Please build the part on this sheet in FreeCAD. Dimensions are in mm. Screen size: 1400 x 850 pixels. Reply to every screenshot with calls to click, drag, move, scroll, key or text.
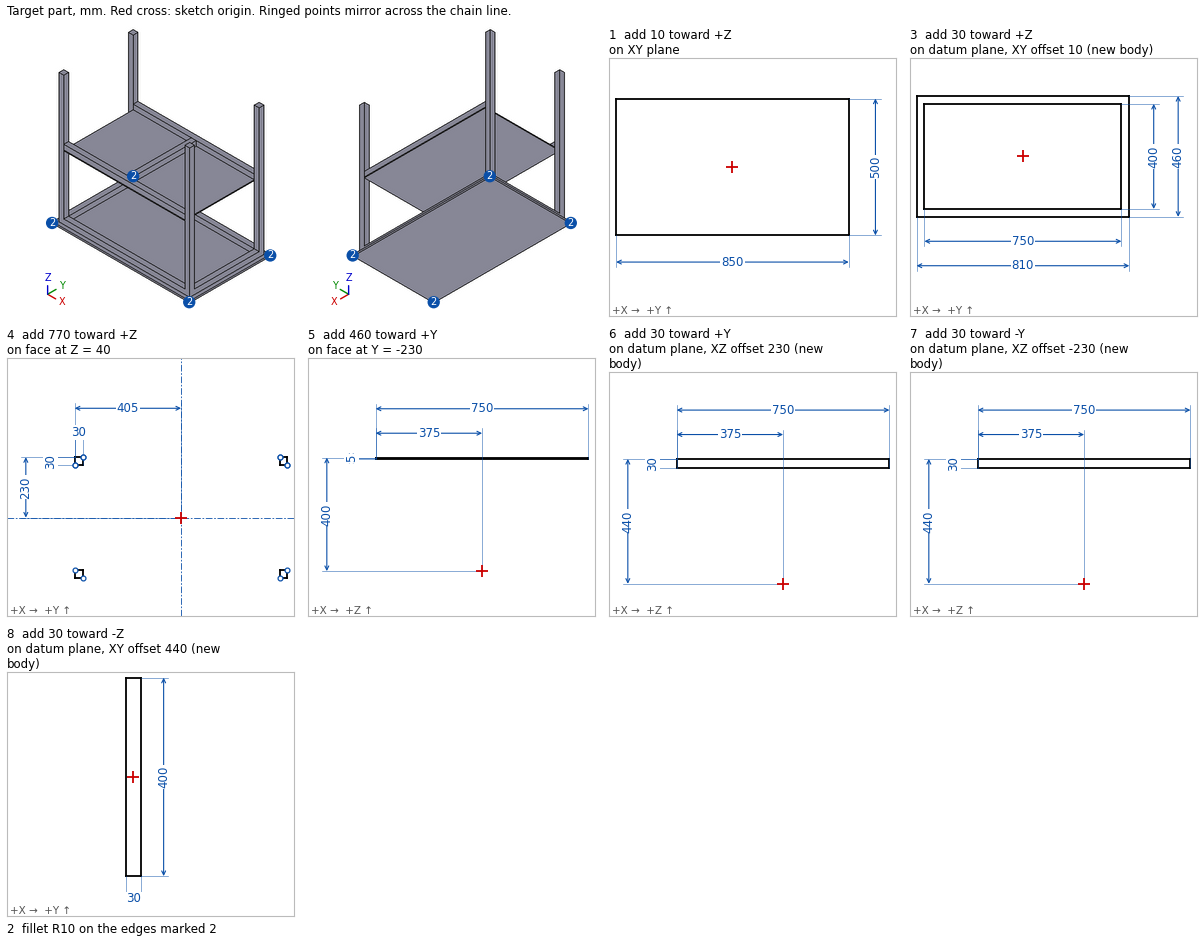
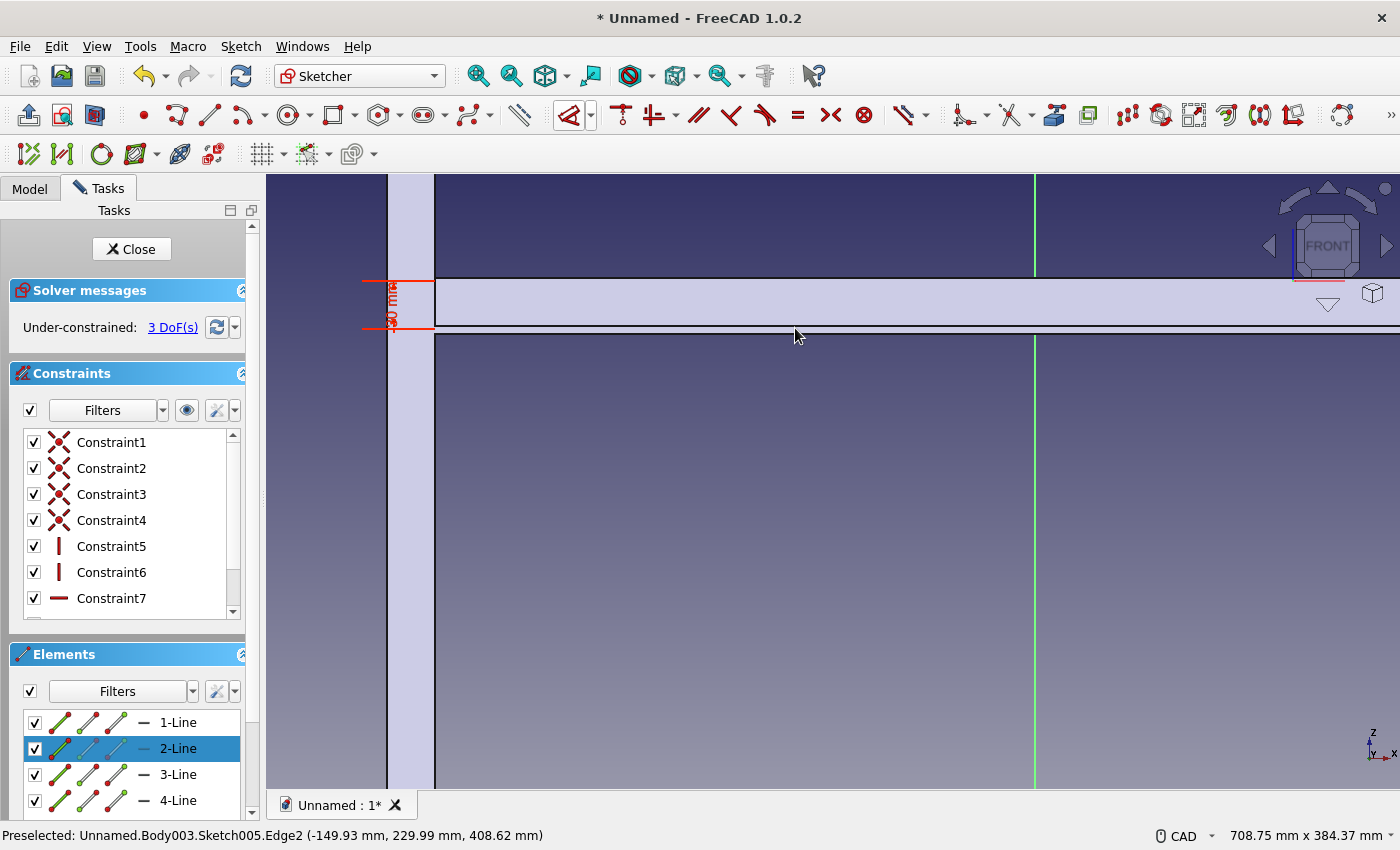
click(590, 116)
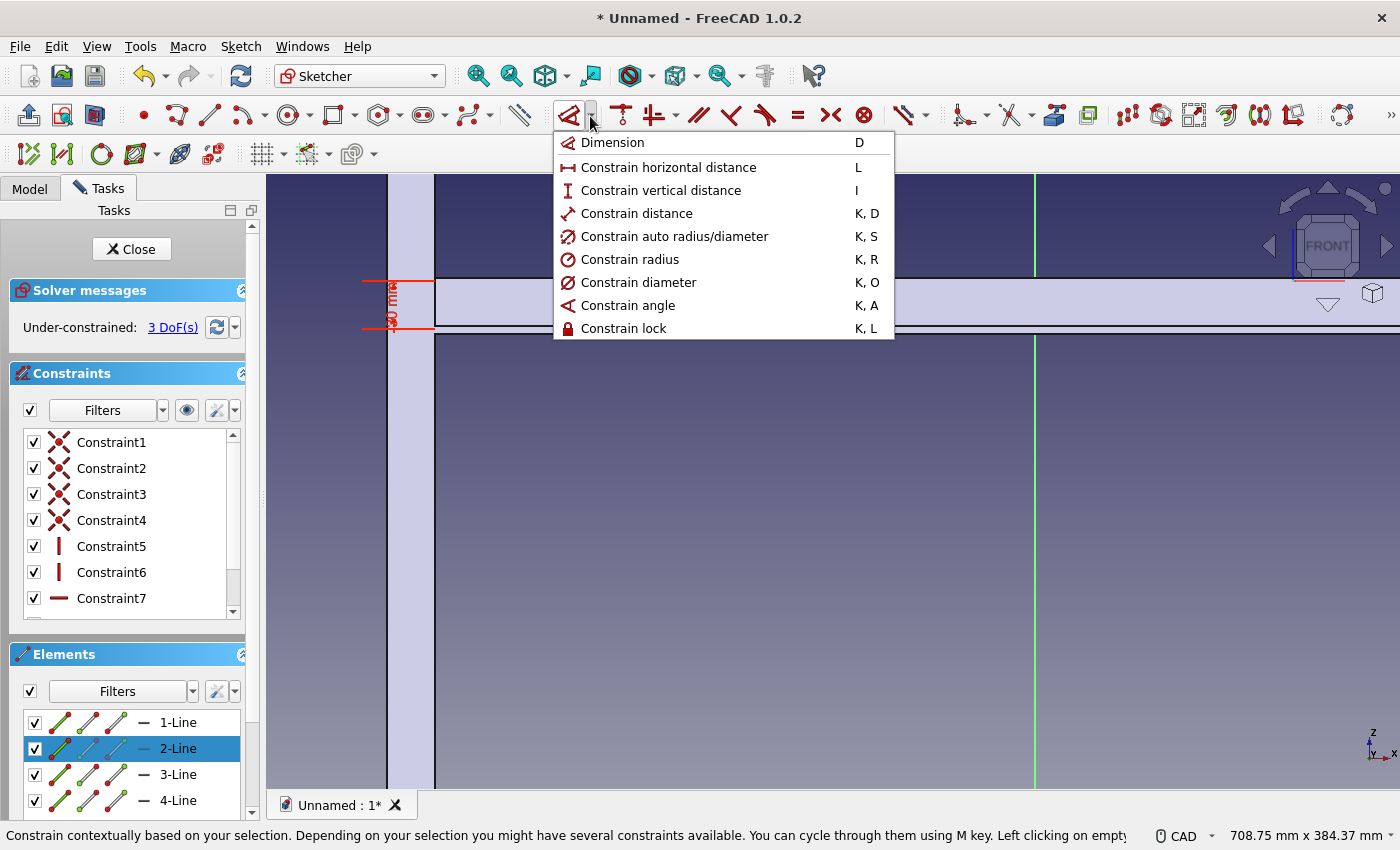
click(724, 168)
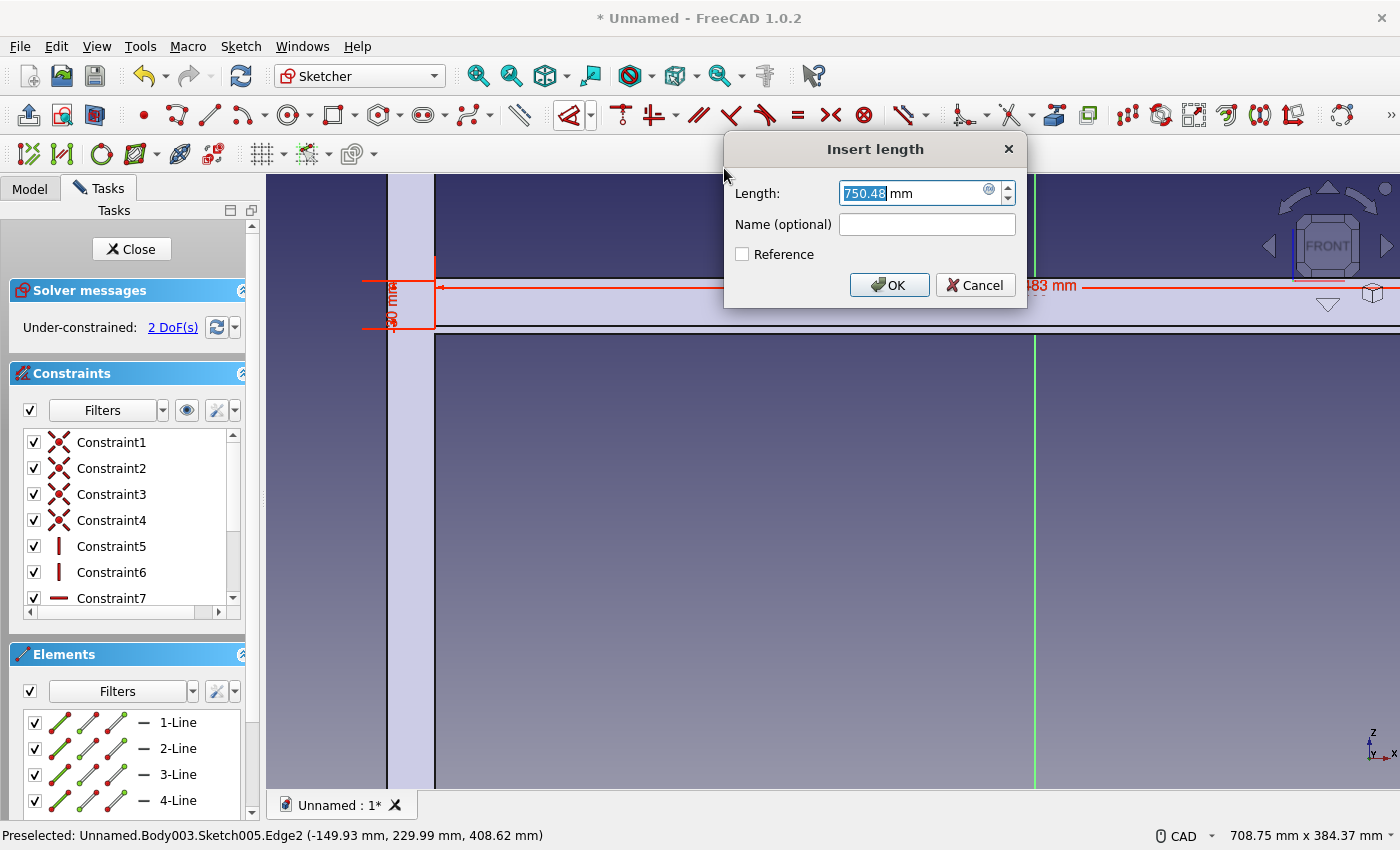
text(750)
key(Return)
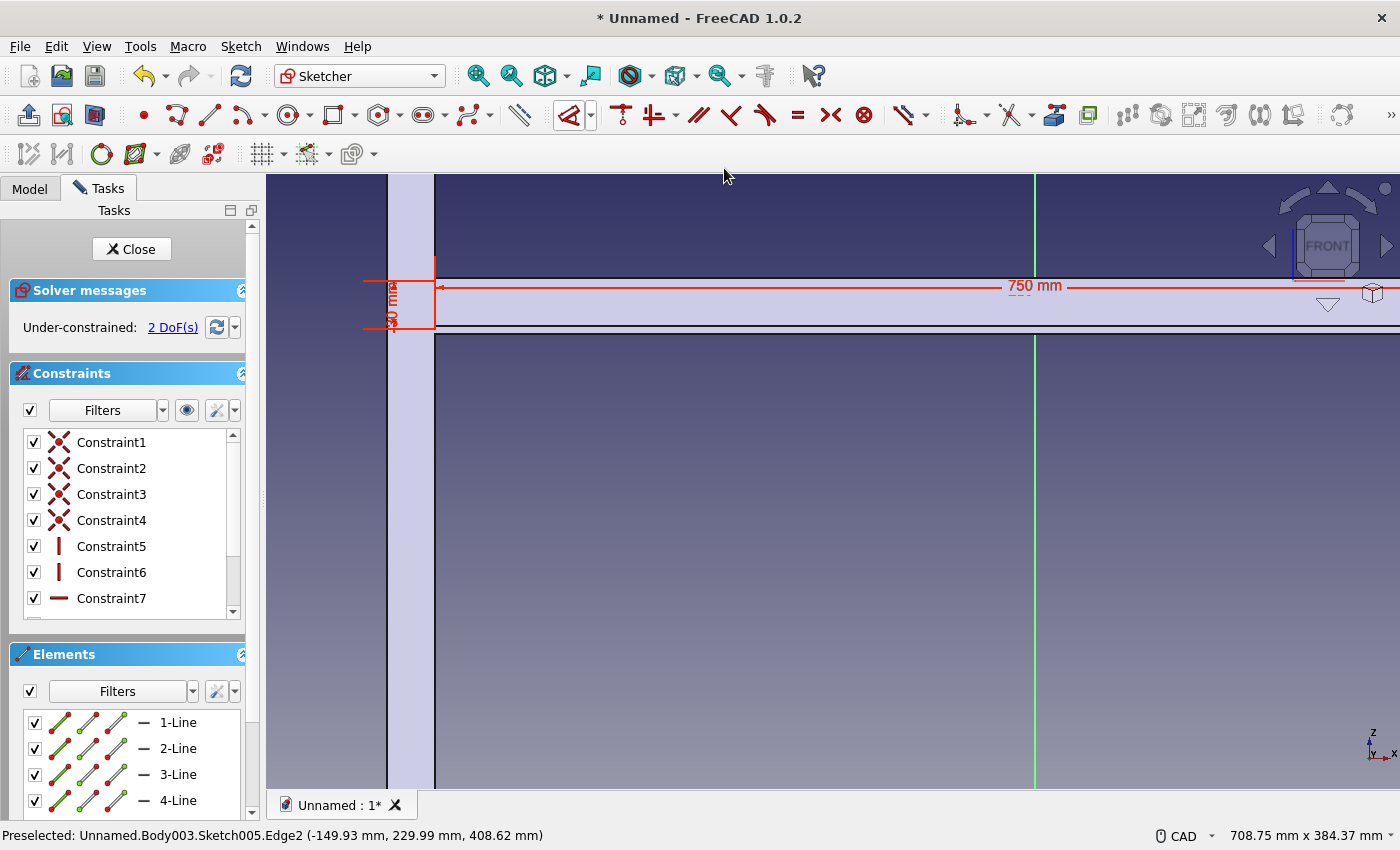
click(435, 280)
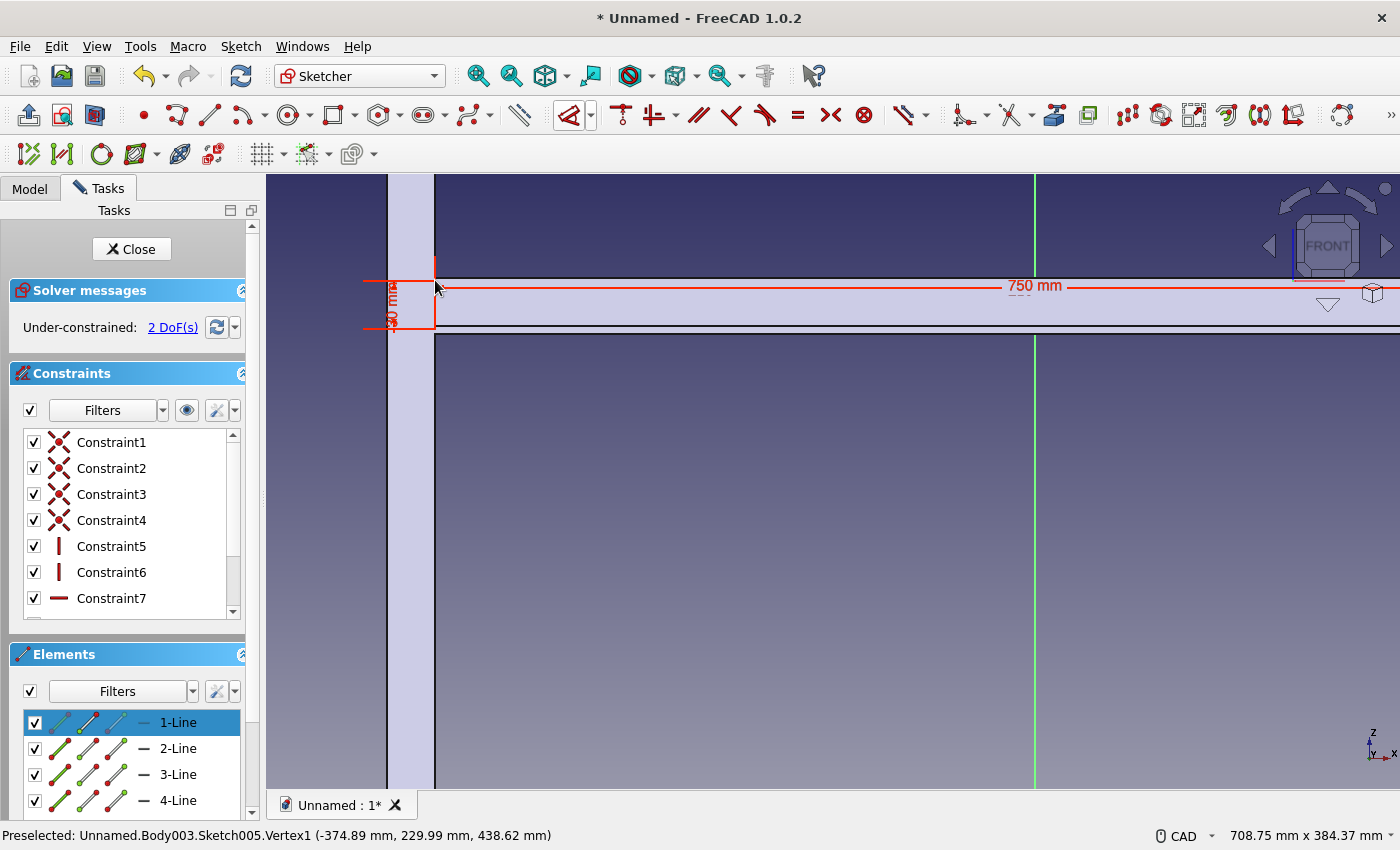
click(590, 116)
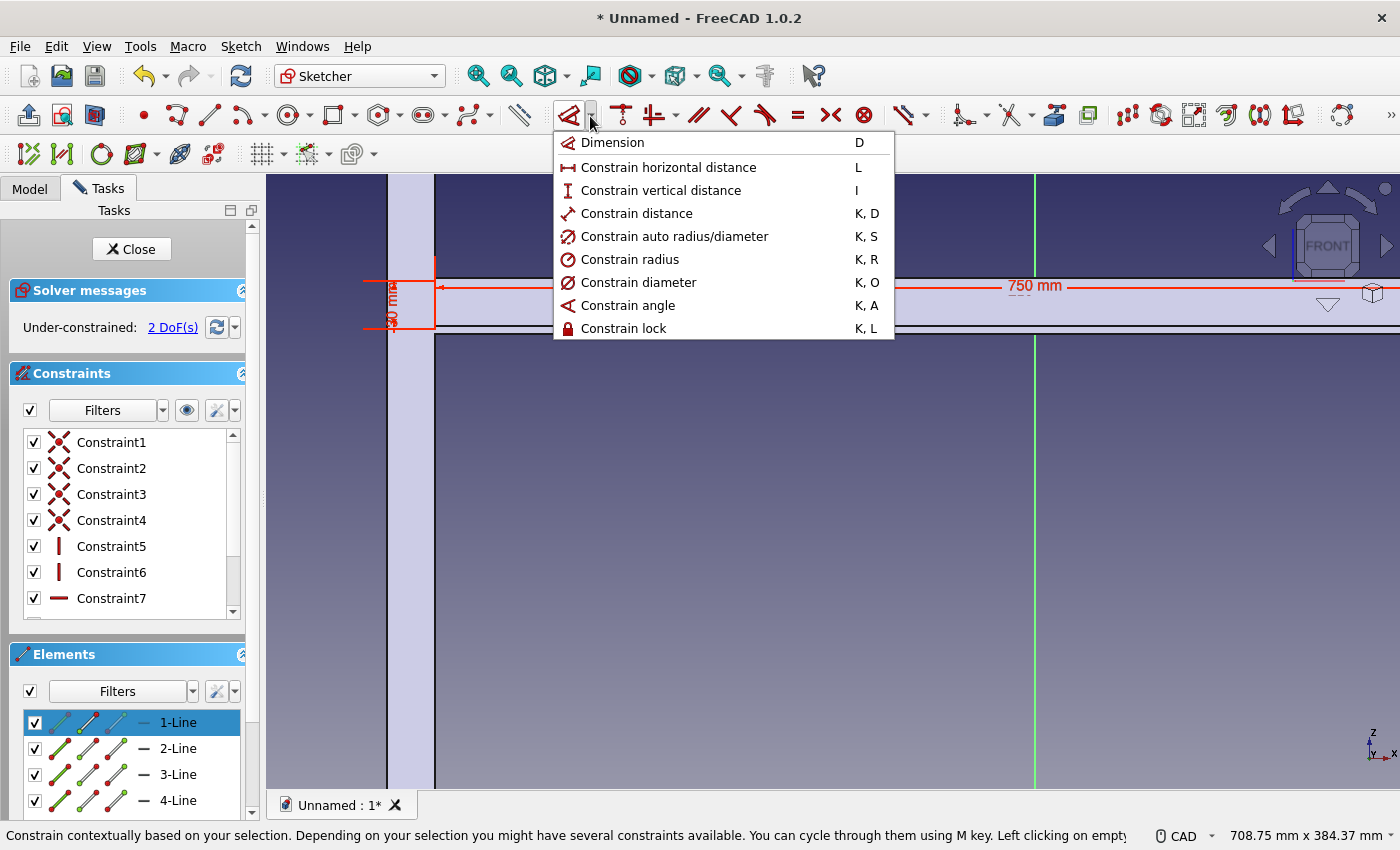
click(724, 168)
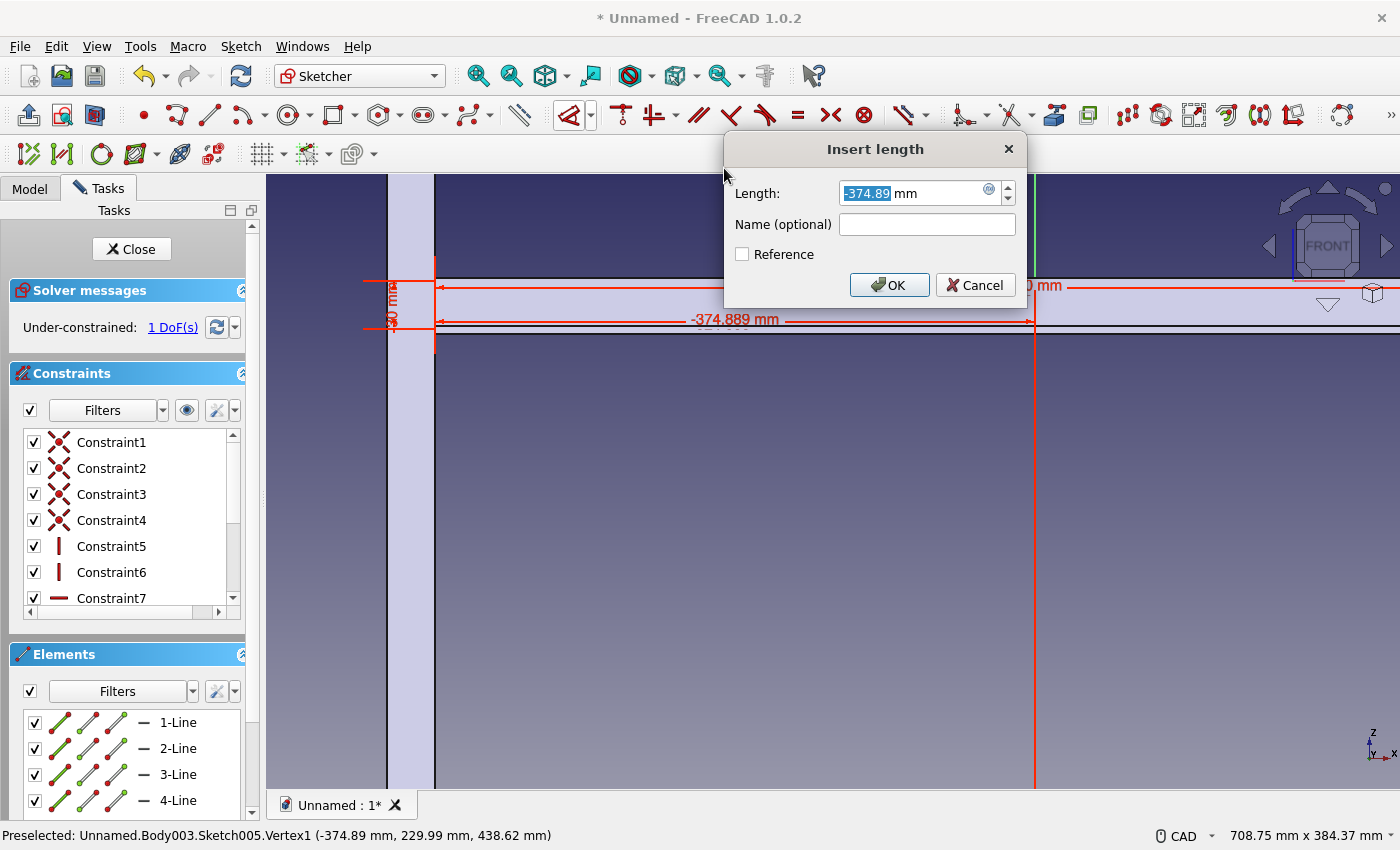
text(-375)
key(Return)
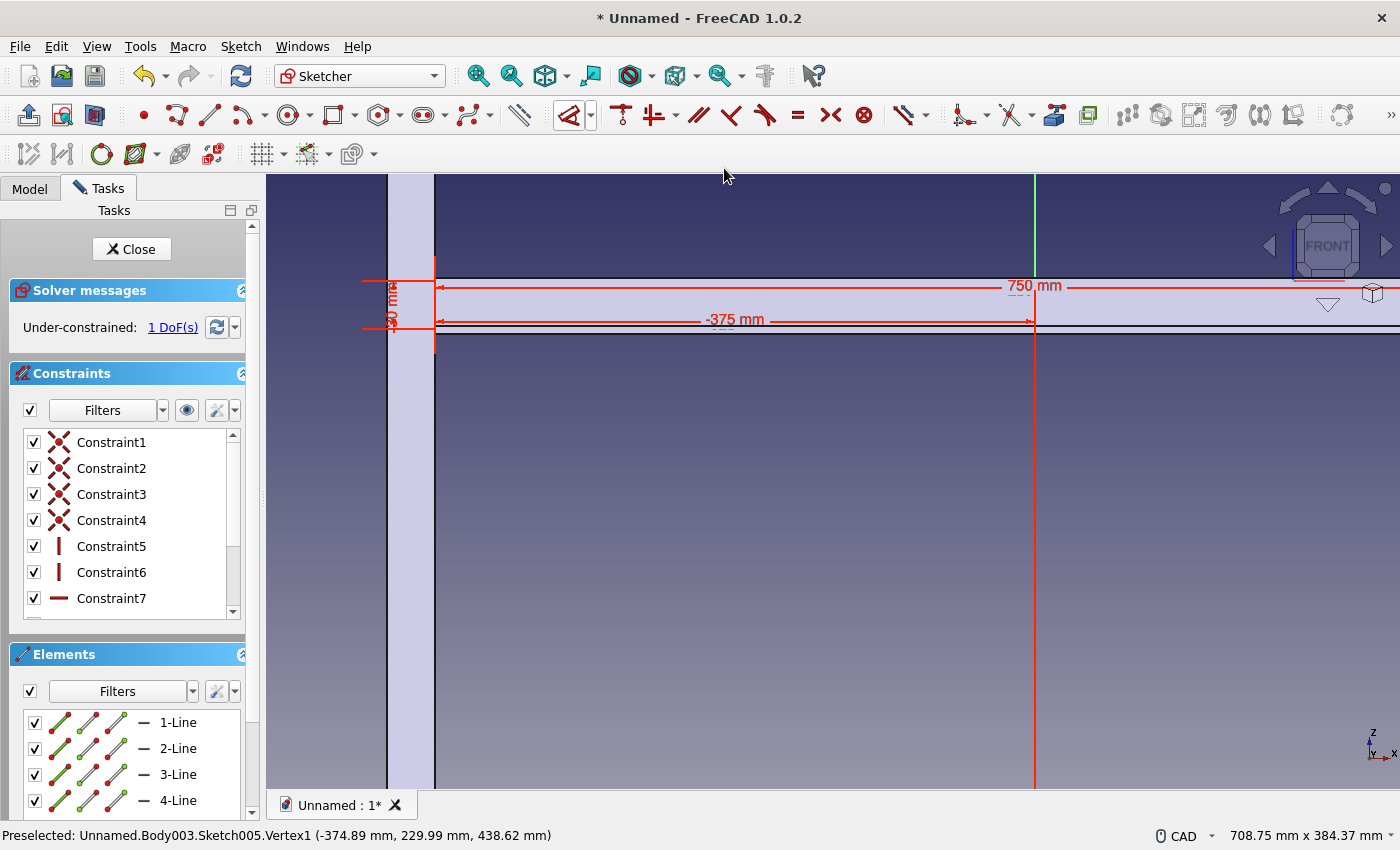
click(435, 280)